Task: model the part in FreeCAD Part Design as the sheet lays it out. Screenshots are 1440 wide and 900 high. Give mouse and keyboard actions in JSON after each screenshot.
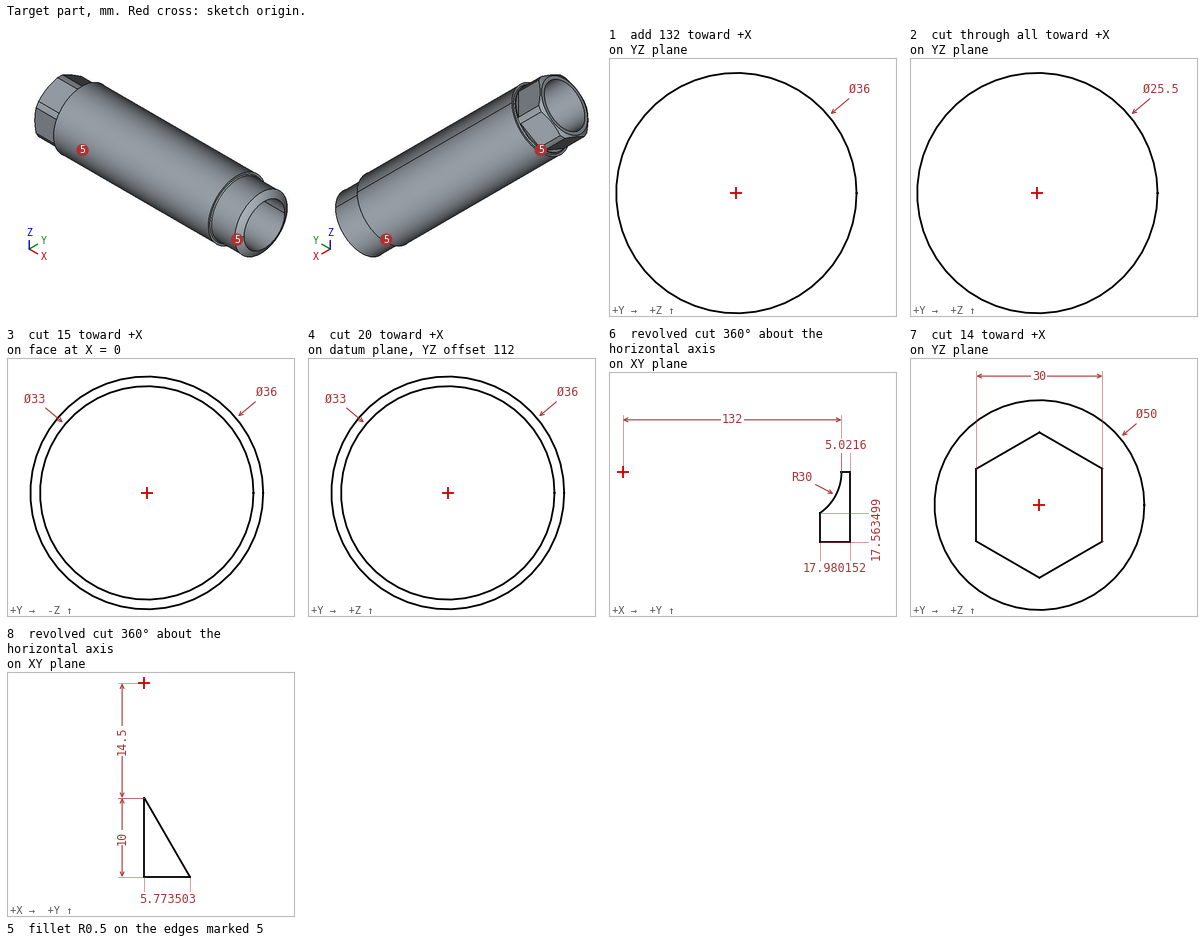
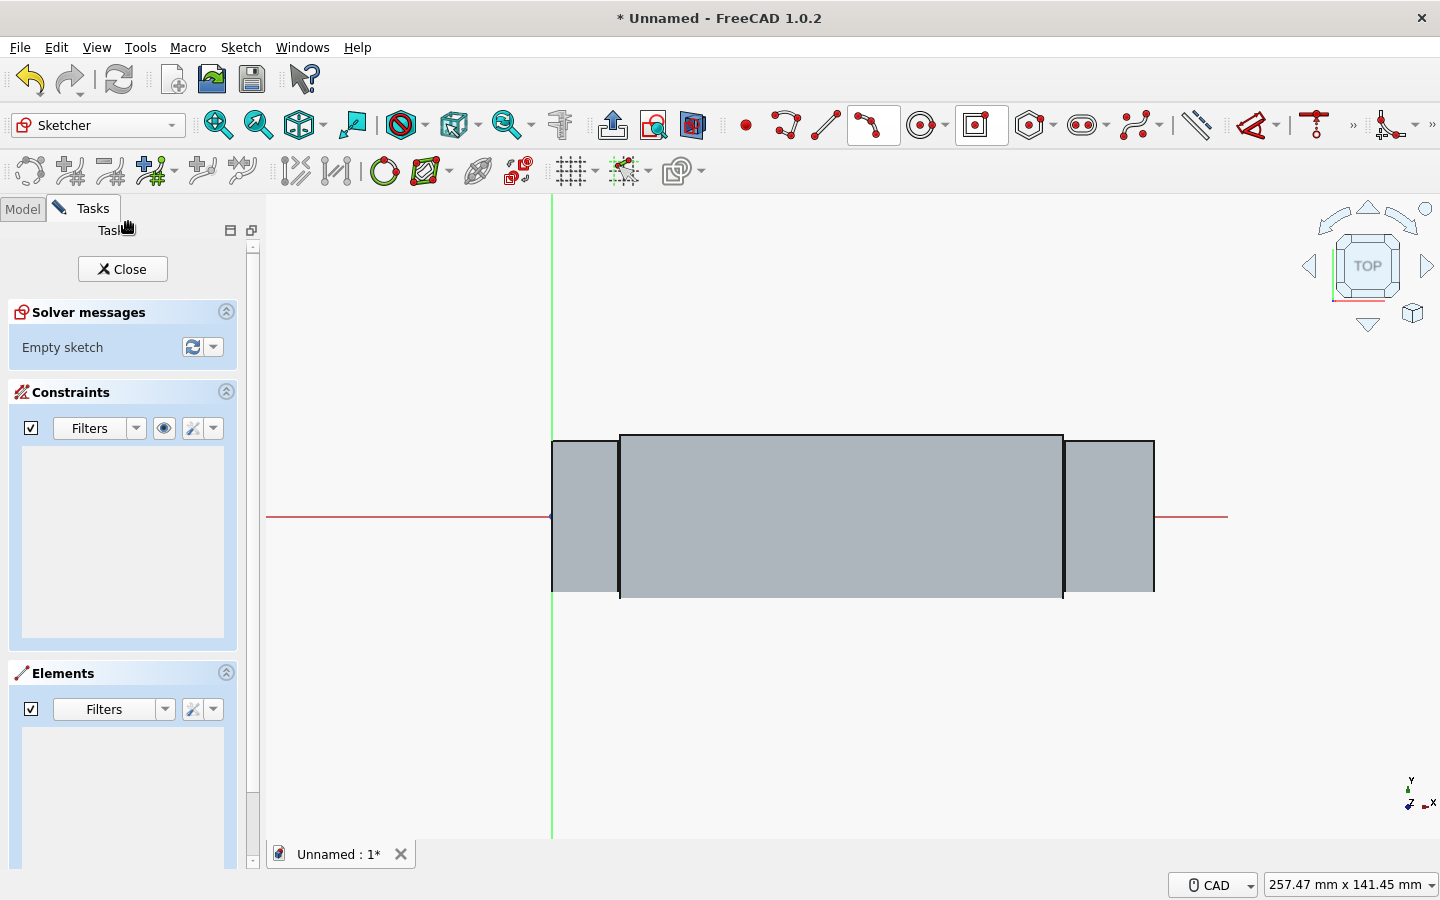
{"action": "key", "text": "q s"}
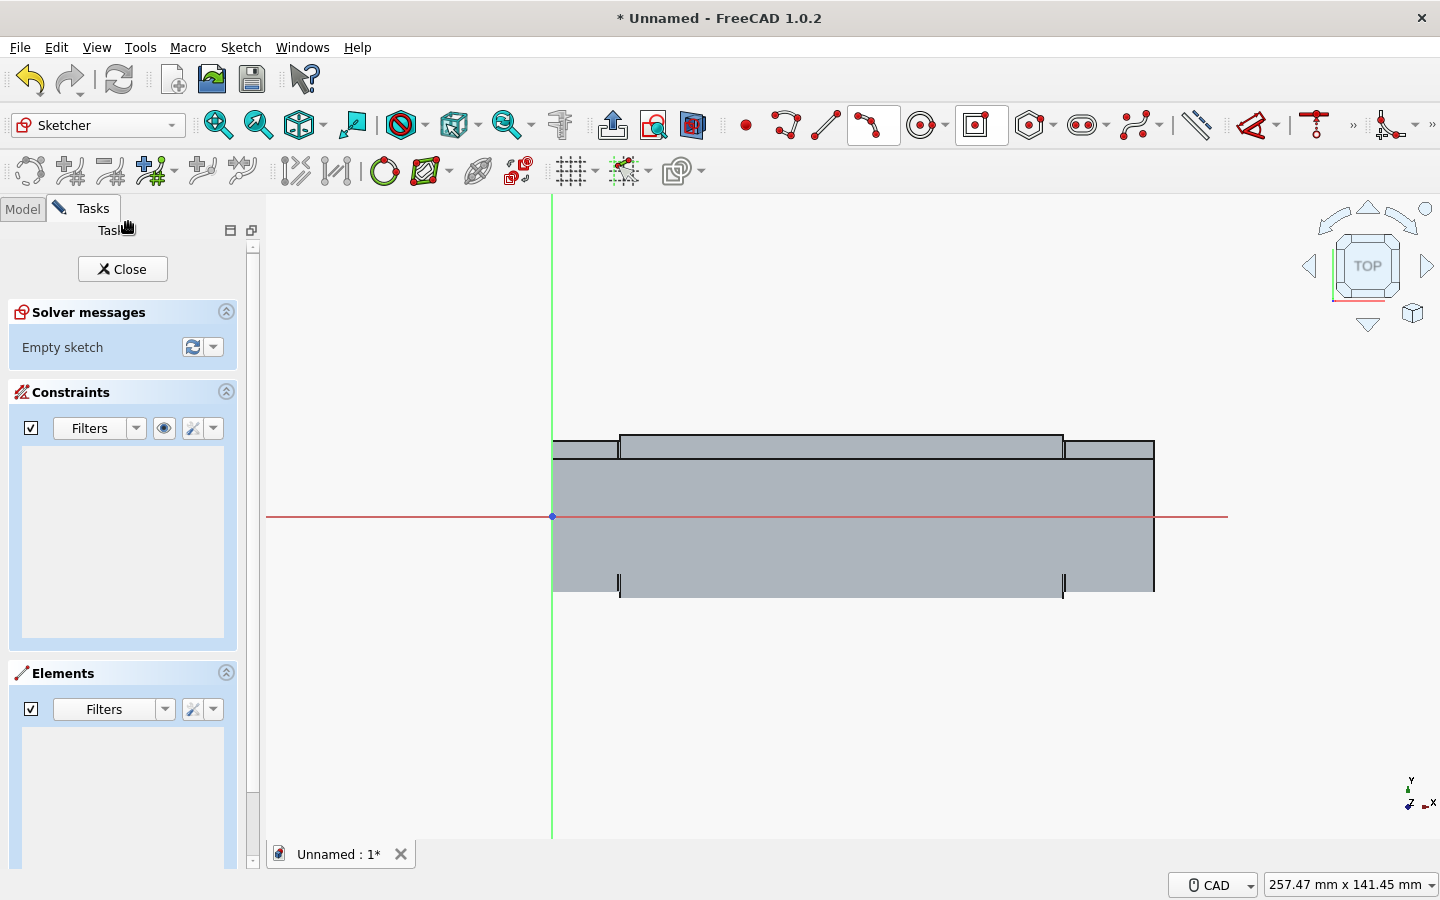
{"action": "scroll", "coordinate": [1275, 692], "scroll_direction": "up", "scroll_amount": 4}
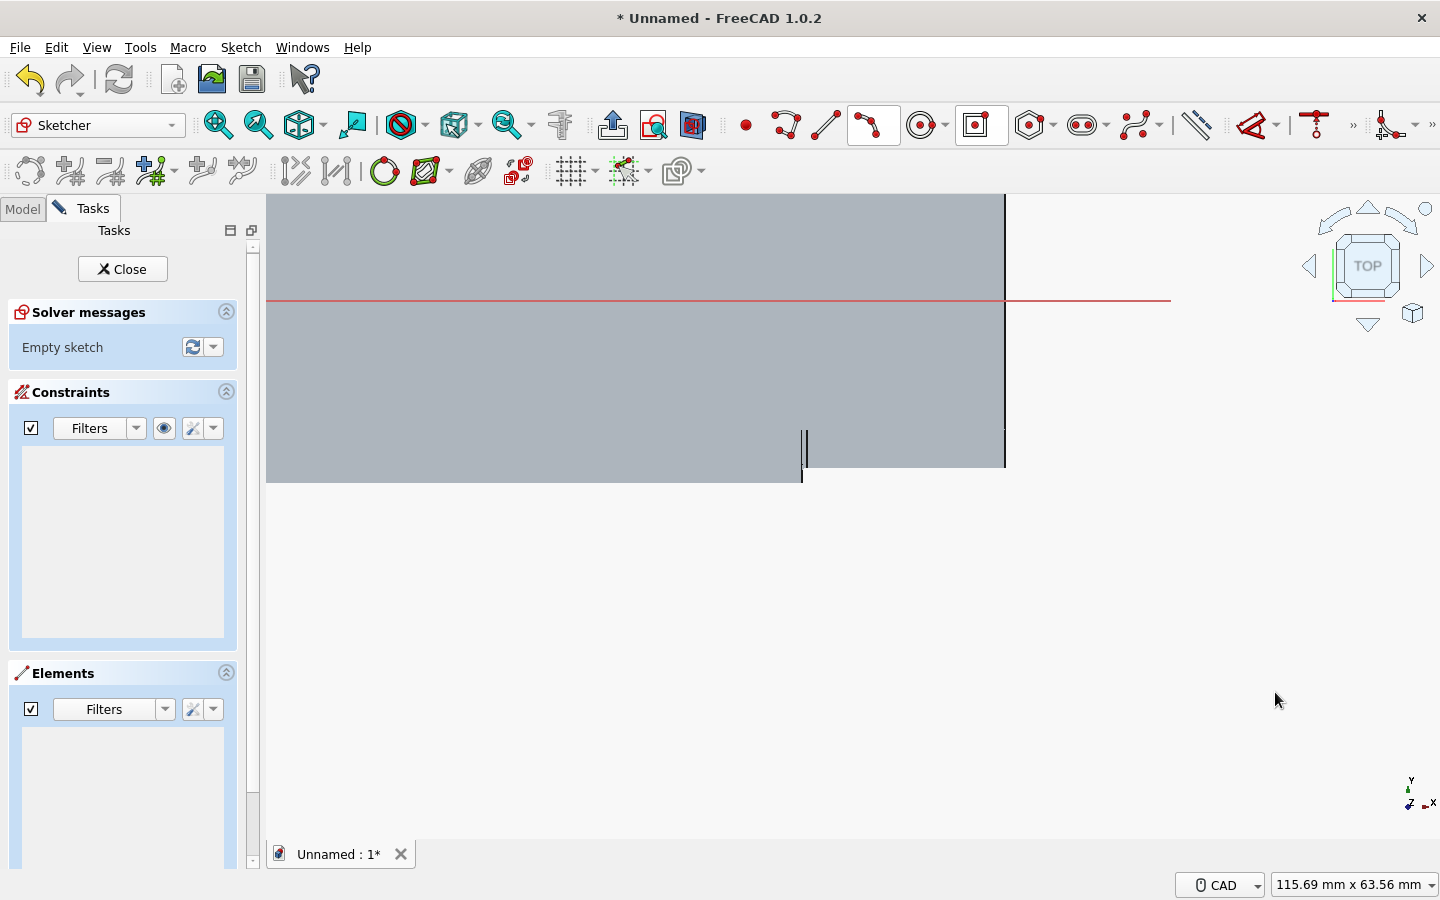
{"action": "left_click", "coordinate": [786, 126]}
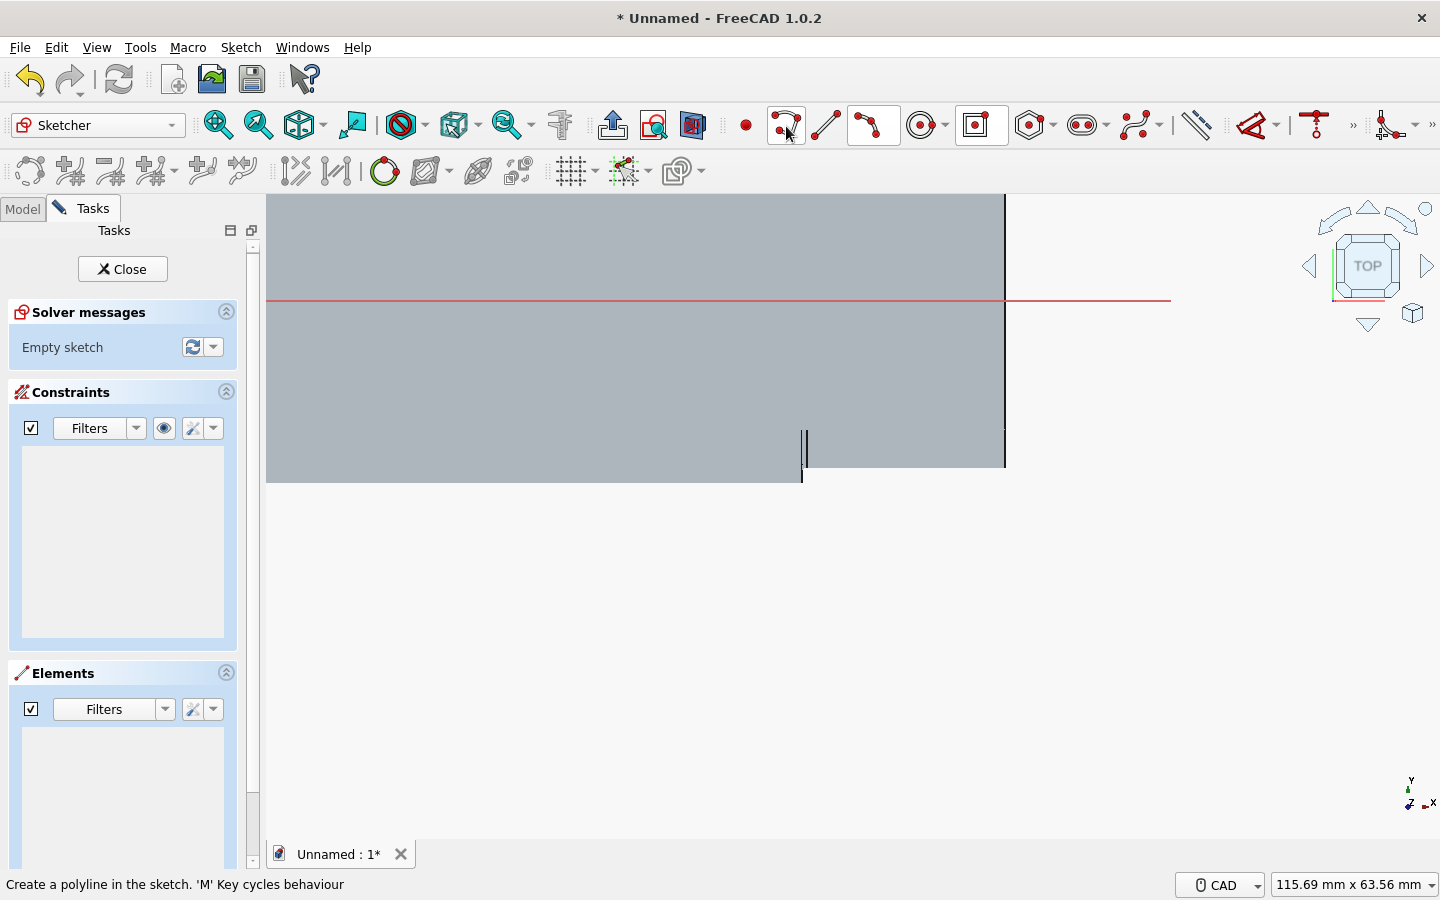
{"action": "left_click", "coordinate": [873, 551]}
{"action": "left_click", "coordinate": [873, 730]}
{"action": "left_click", "coordinate": [1055, 730]}
{"action": "left_click", "coordinate": [1055, 301]}
{"action": "left_click", "coordinate": [1005, 310]}
{"action": "right_click", "coordinate": [1005, 310]}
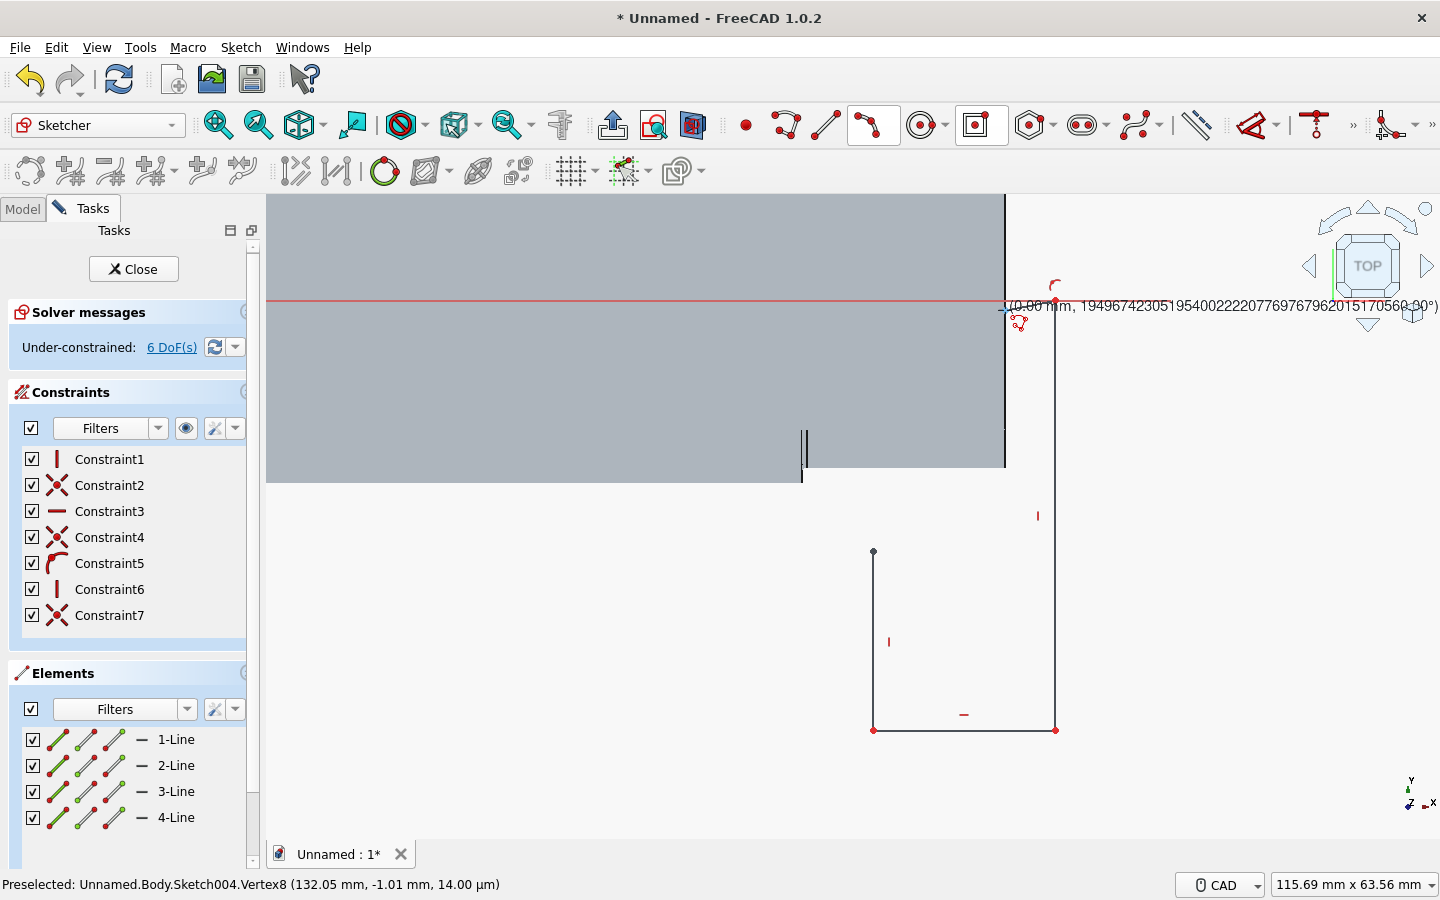
{"action": "left_click", "coordinate": [868, 126]}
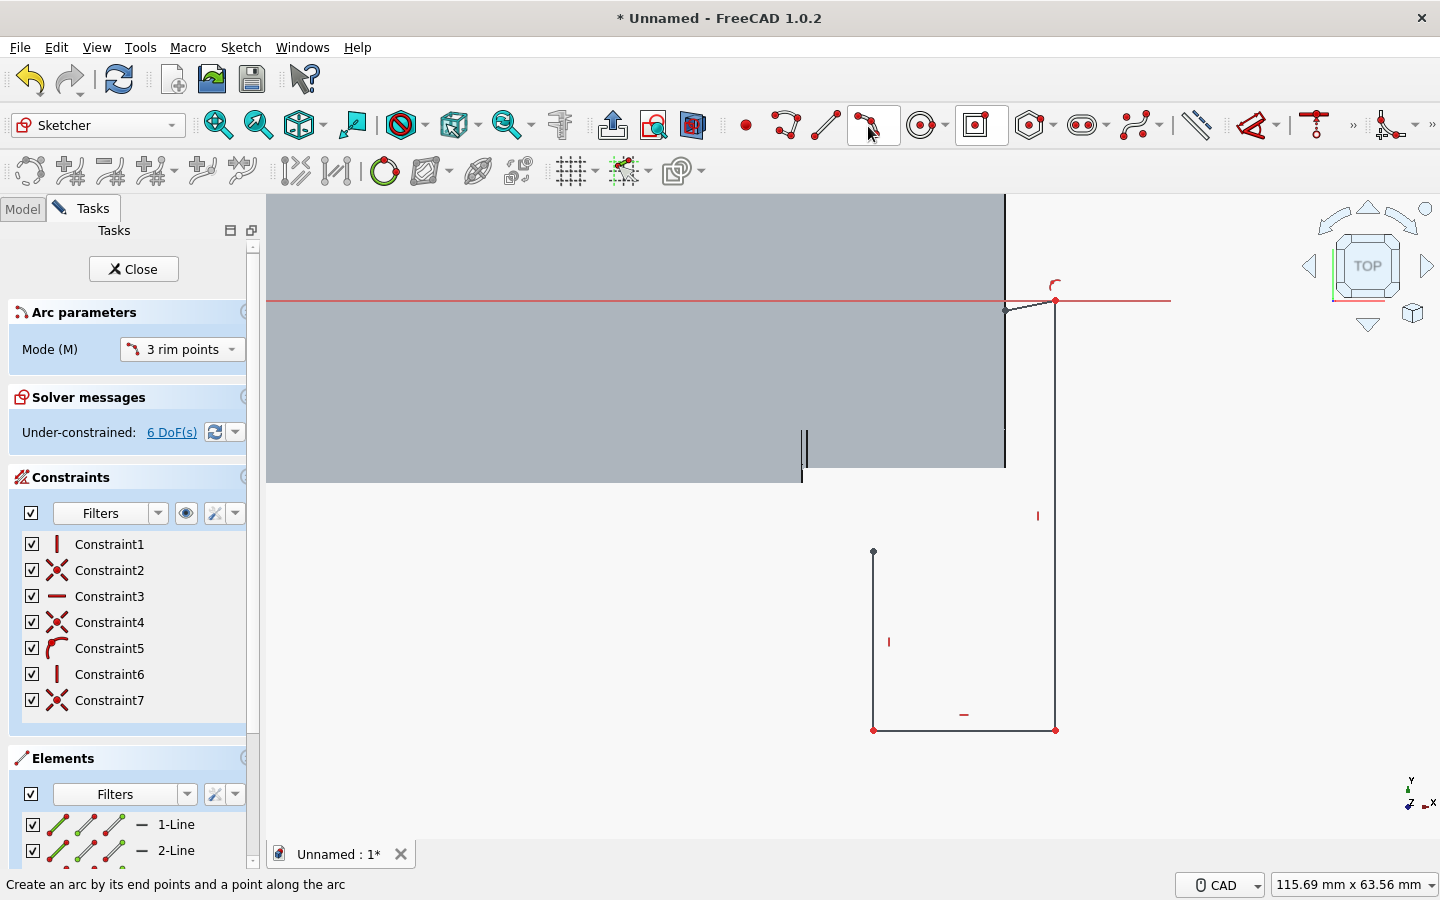
{"action": "left_click", "coordinate": [1005, 311]}
{"action": "left_click", "coordinate": [873, 552]}
{"action": "left_click", "coordinate": [970, 442]}
{"action": "key", "text": "Escape"}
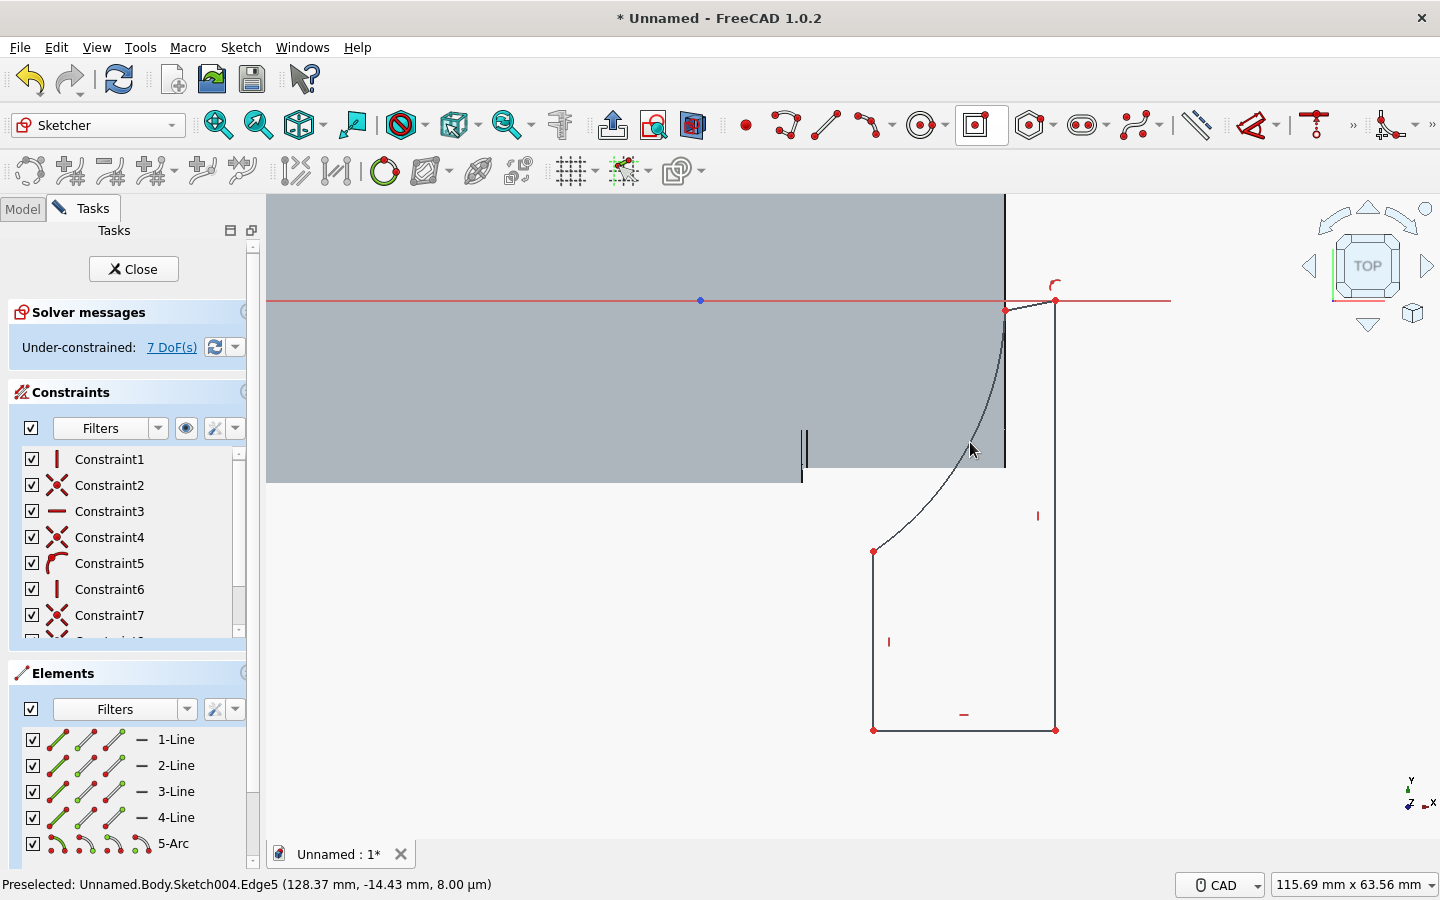
{"action": "left_click", "coordinate": [1040, 304]}